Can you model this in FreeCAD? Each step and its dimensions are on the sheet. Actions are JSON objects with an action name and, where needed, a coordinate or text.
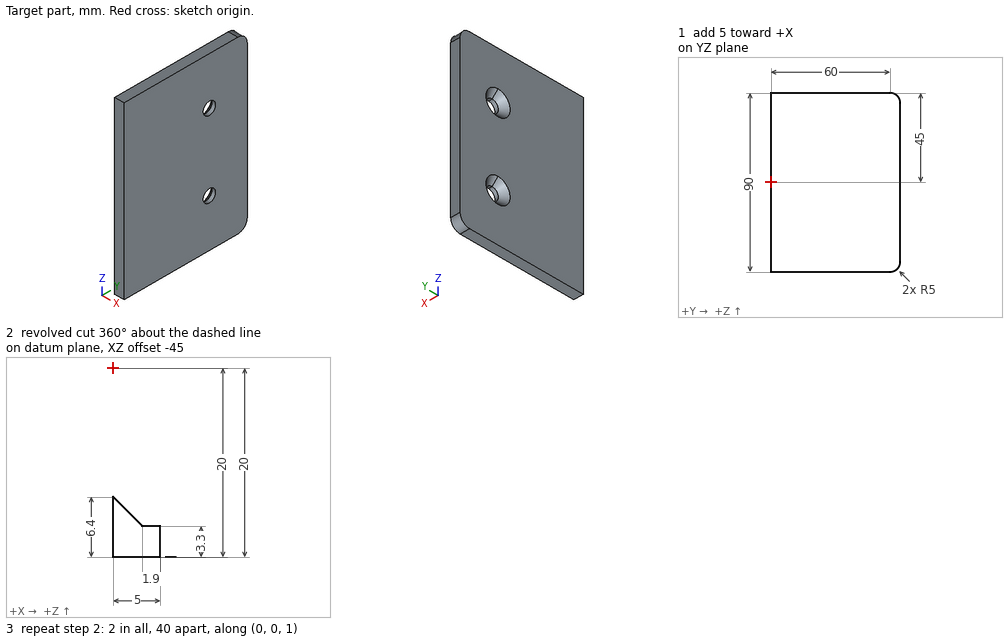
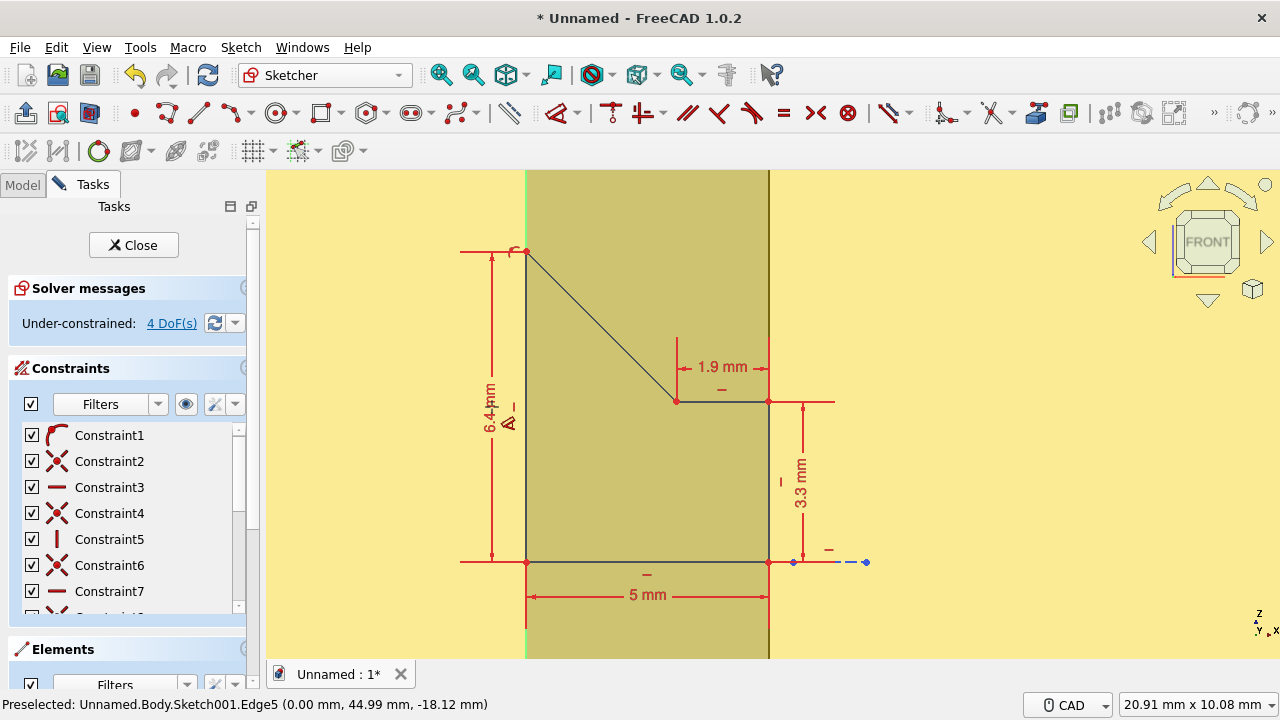
{"action": "left_click", "coordinate": [769, 562]}
{"action": "left_click", "coordinate": [492, 380]}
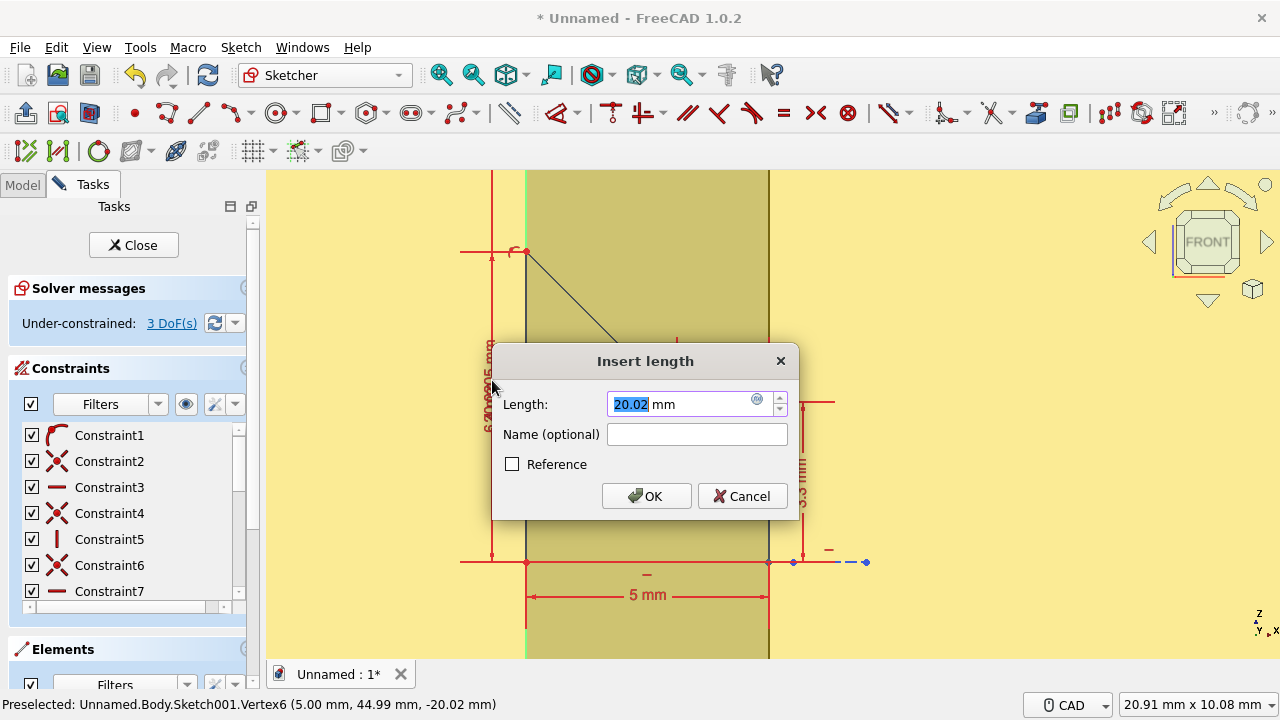
{"action": "type", "text": "20"}
{"action": "key", "text": "Return"}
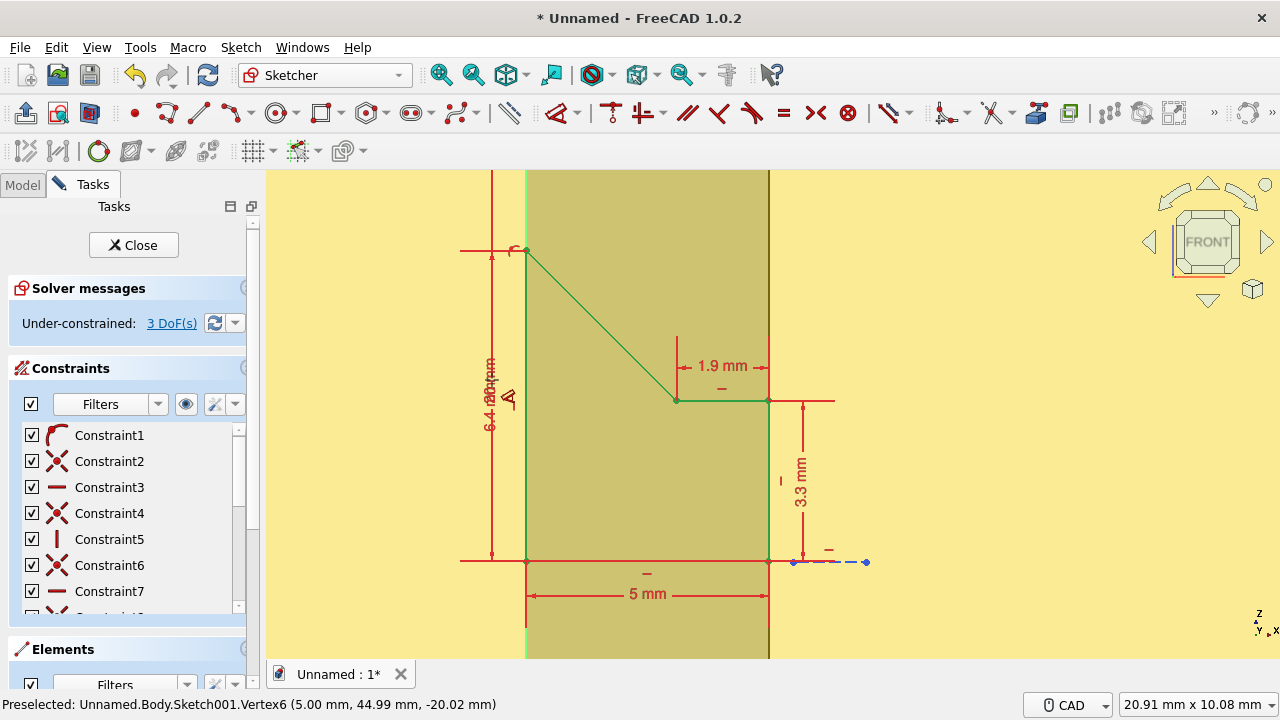
{"action": "left_click", "coordinate": [793, 562]}
{"action": "left_click", "coordinate": [492, 296]}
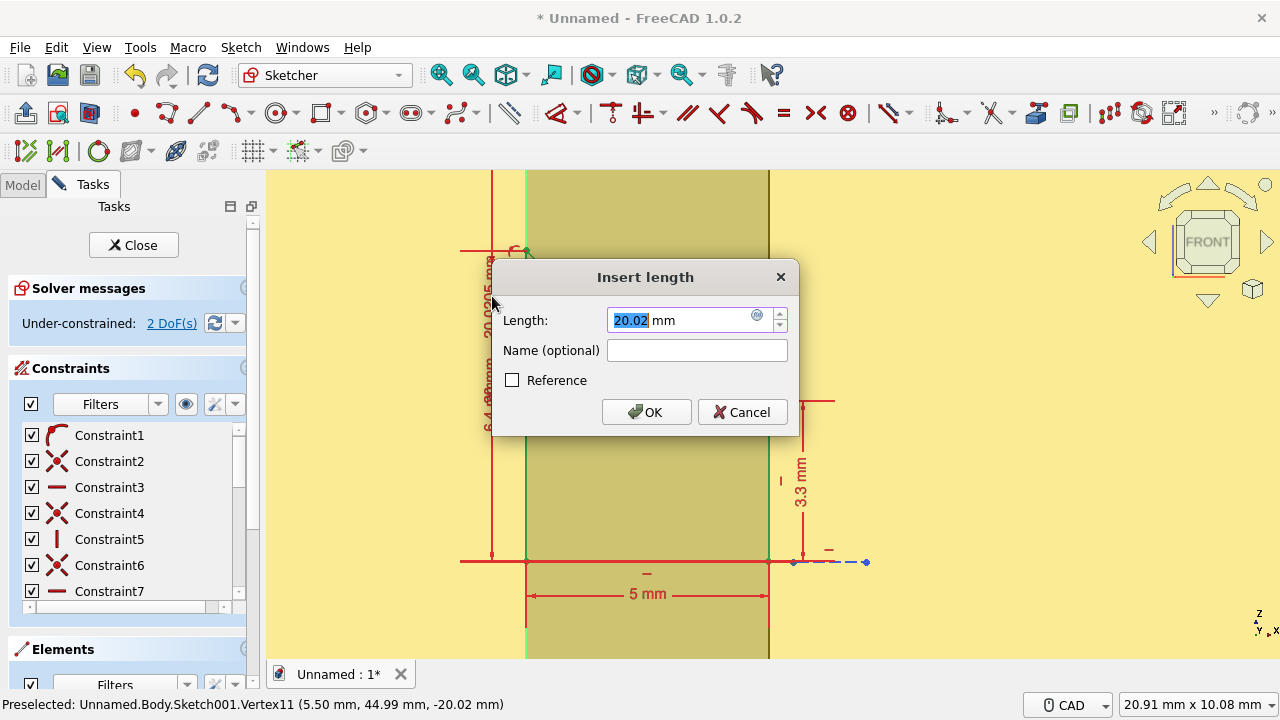
{"action": "type", "text": "20"}
{"action": "key", "text": "Return"}
{"action": "key", "text": "Escape"}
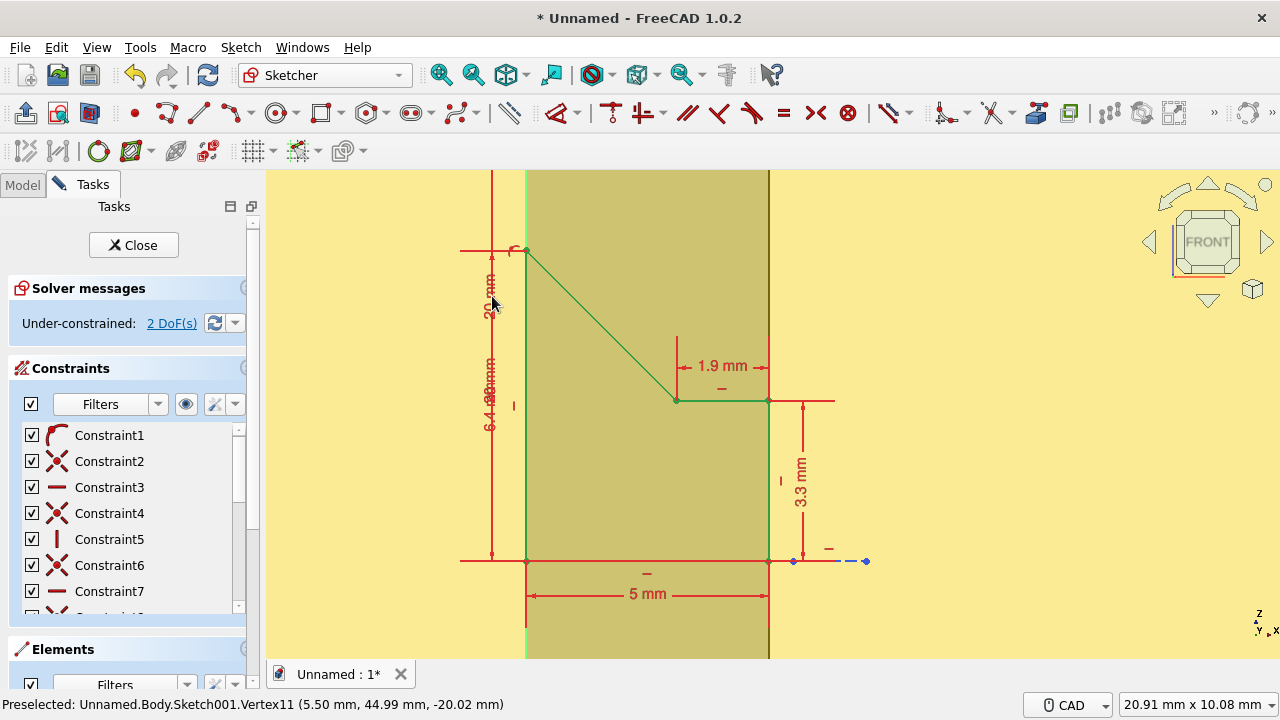
{"action": "left_click", "coordinate": [134, 245]}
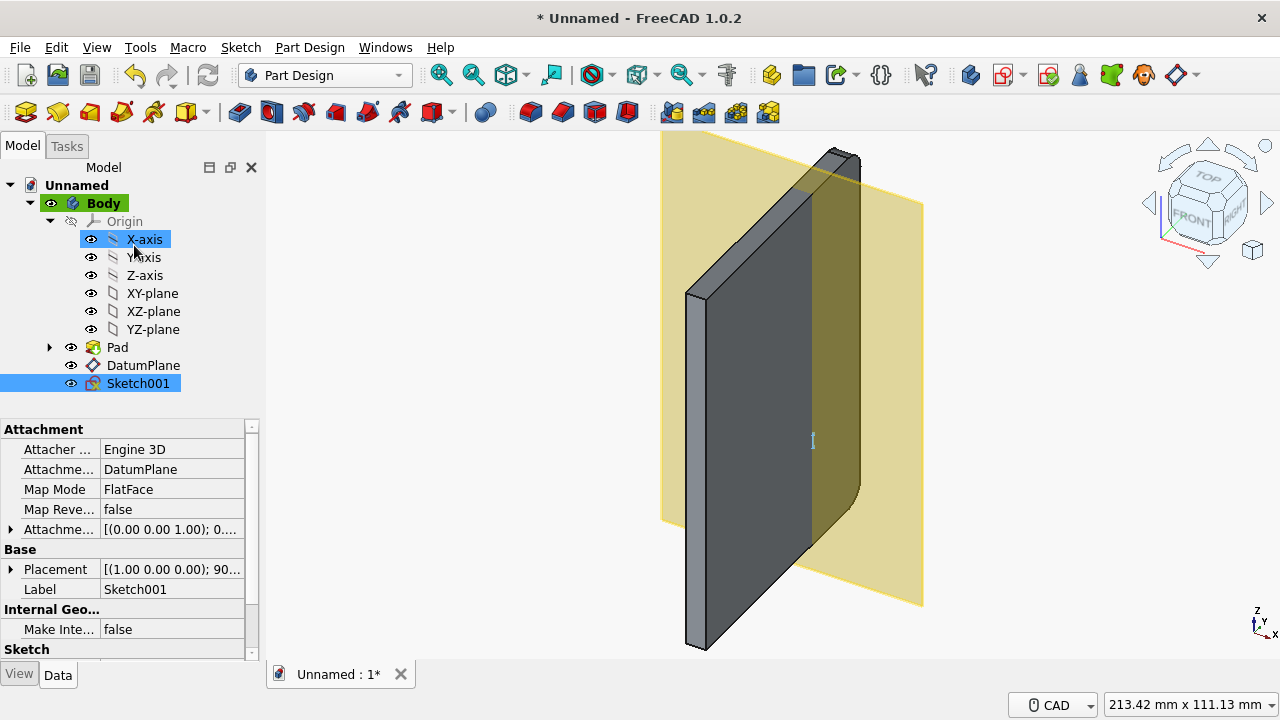
{"action": "left_click", "coordinate": [304, 112]}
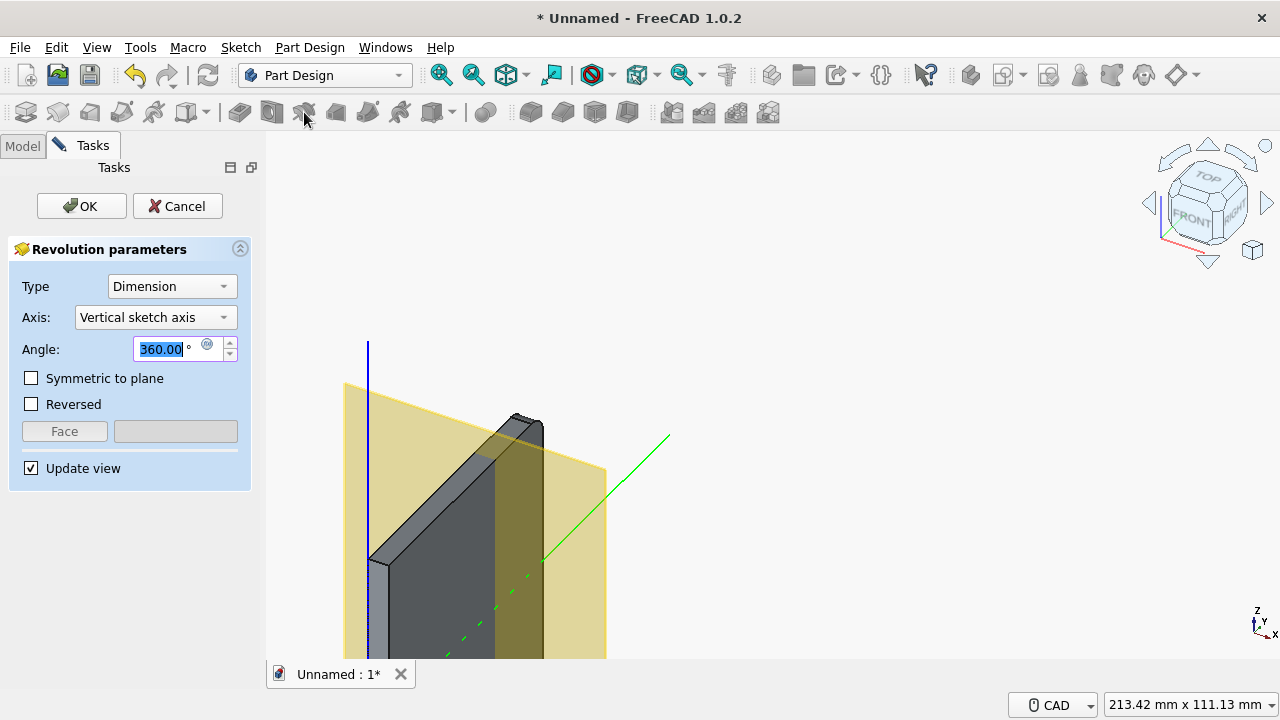
{"action": "left_click", "coordinate": [156, 318]}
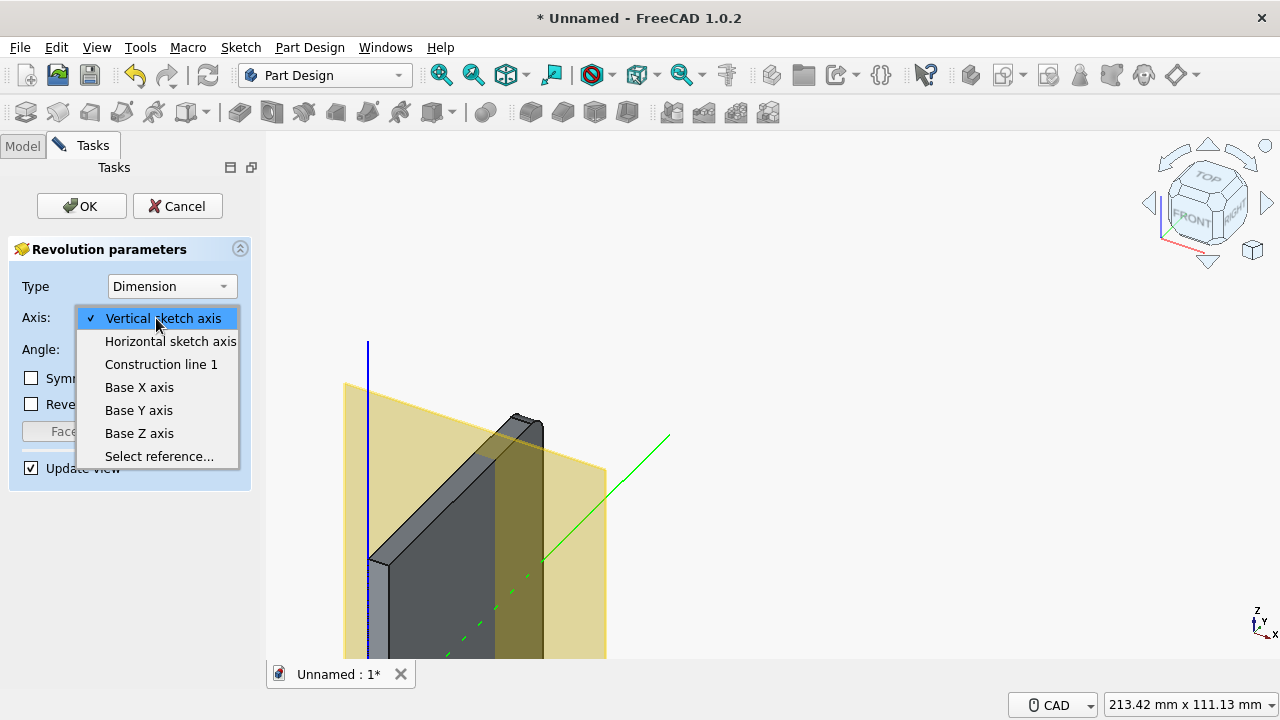
{"action": "left_click", "coordinate": [156, 364]}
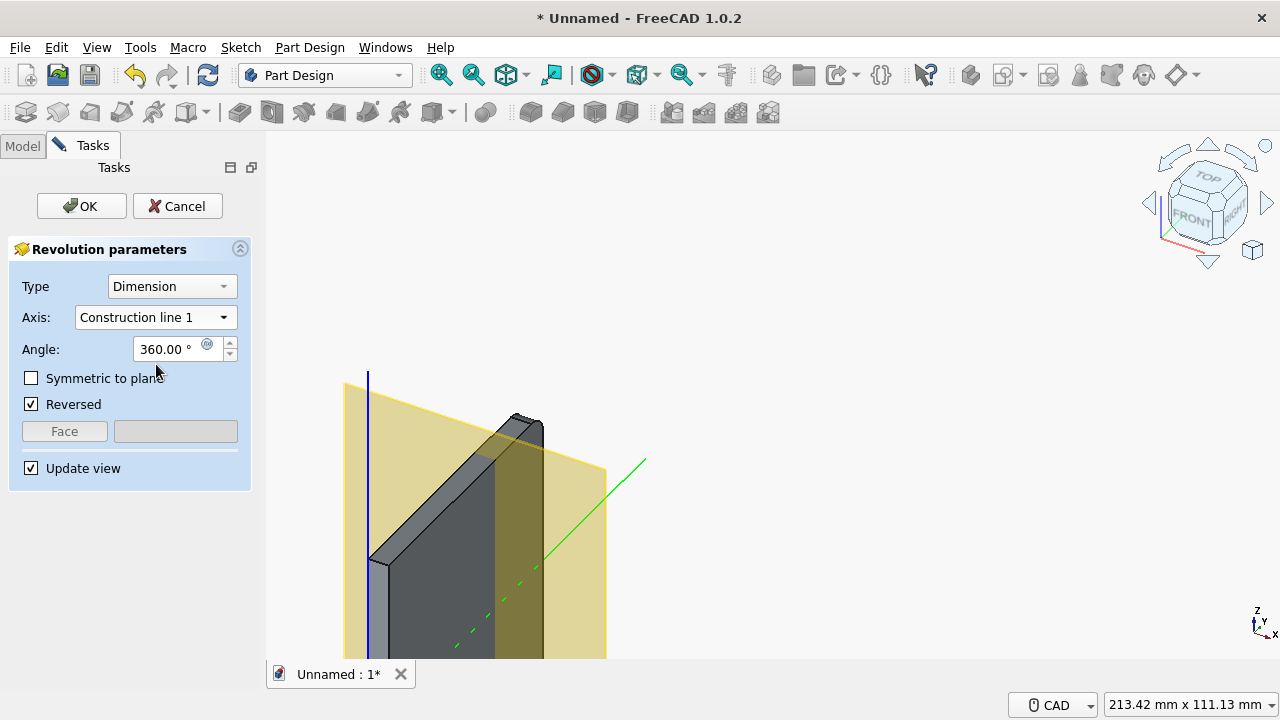
{"action": "left_click", "coordinate": [82, 206]}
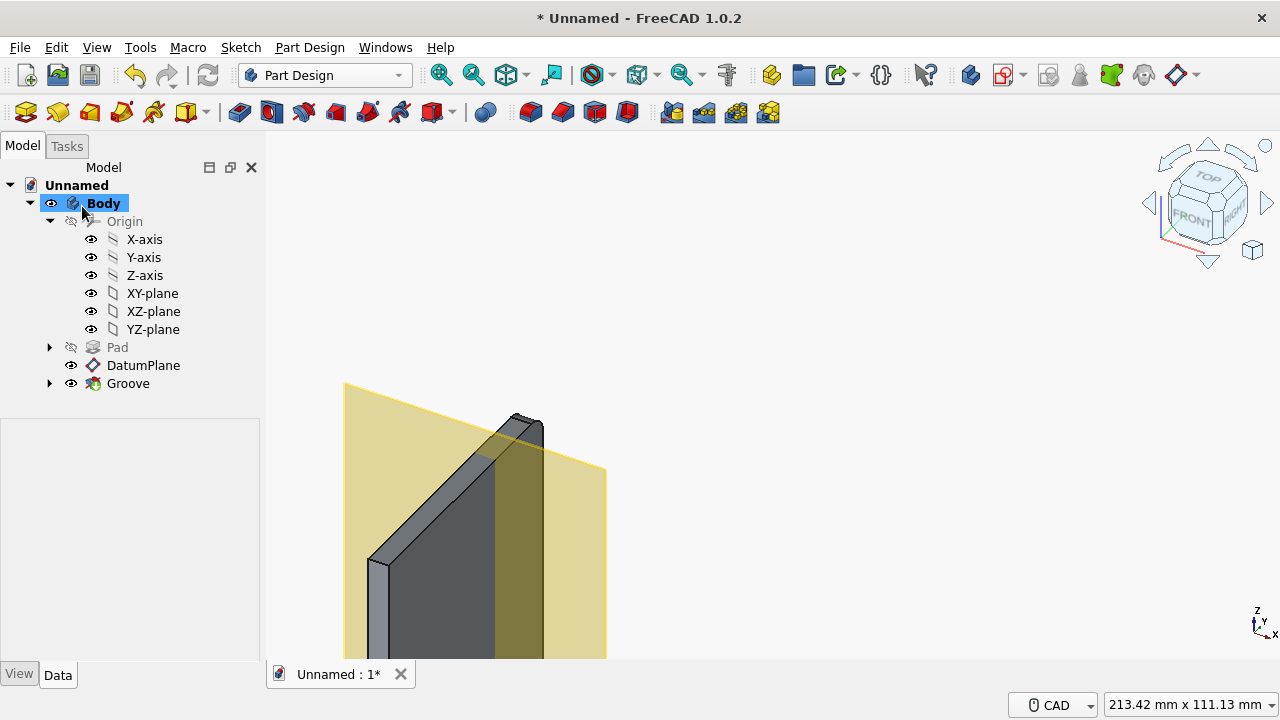
{"action": "left_click", "coordinate": [116, 365]}
{"action": "key", "text": "space"}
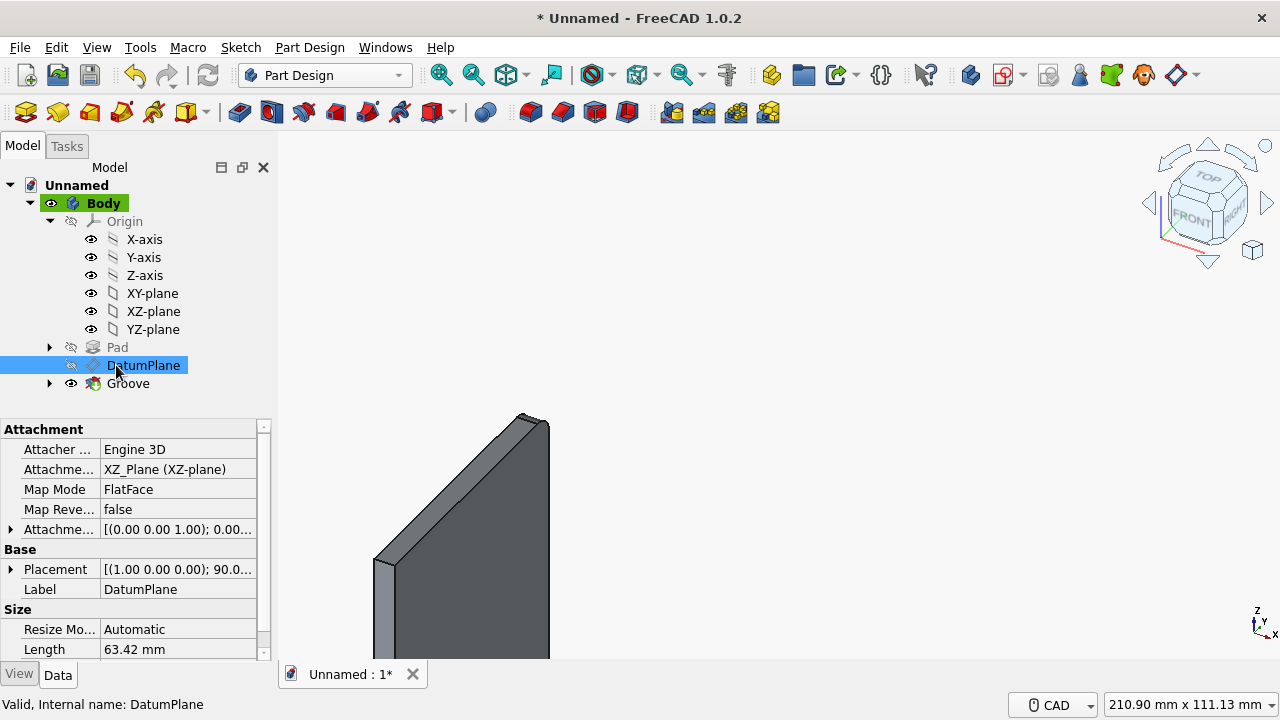
{"action": "left_click", "coordinate": [442, 76]}